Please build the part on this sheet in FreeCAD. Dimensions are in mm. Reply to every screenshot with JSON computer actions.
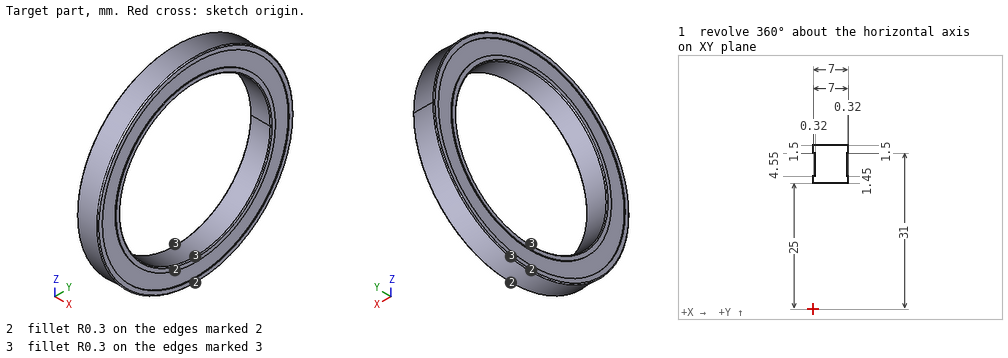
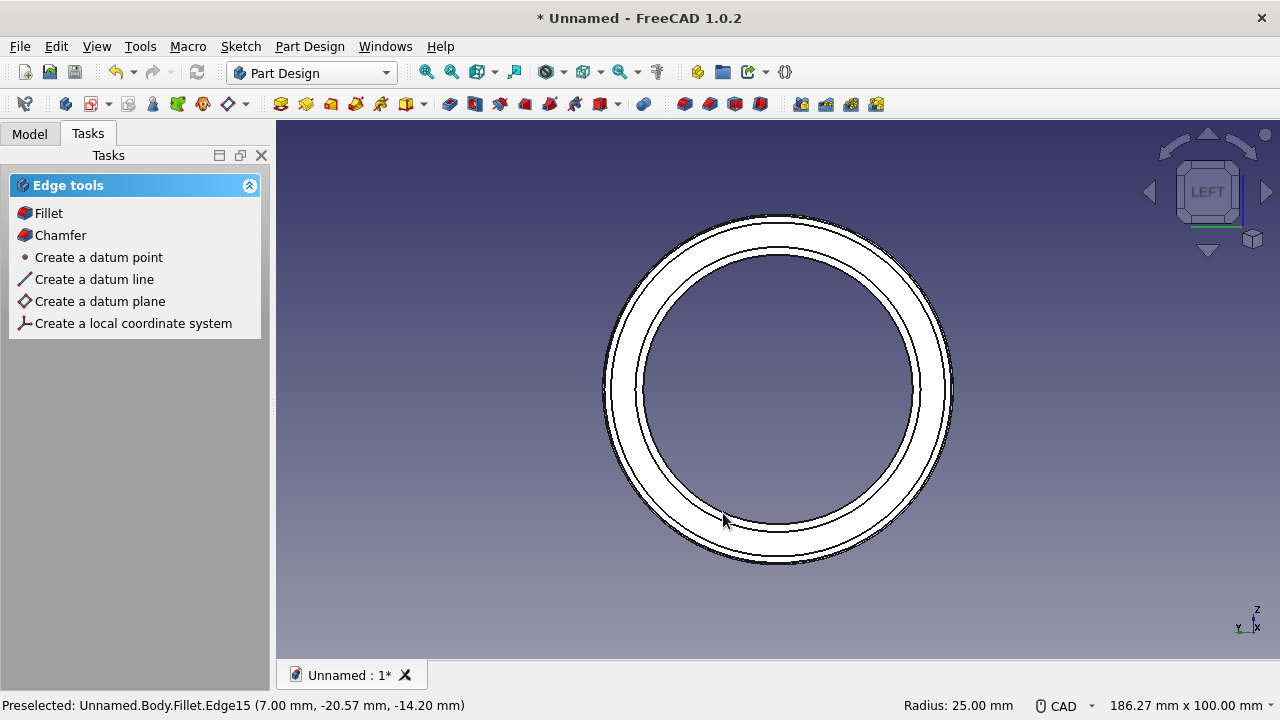
{"action": "left_click", "coordinate": [887, 309], "text": "ctrl"}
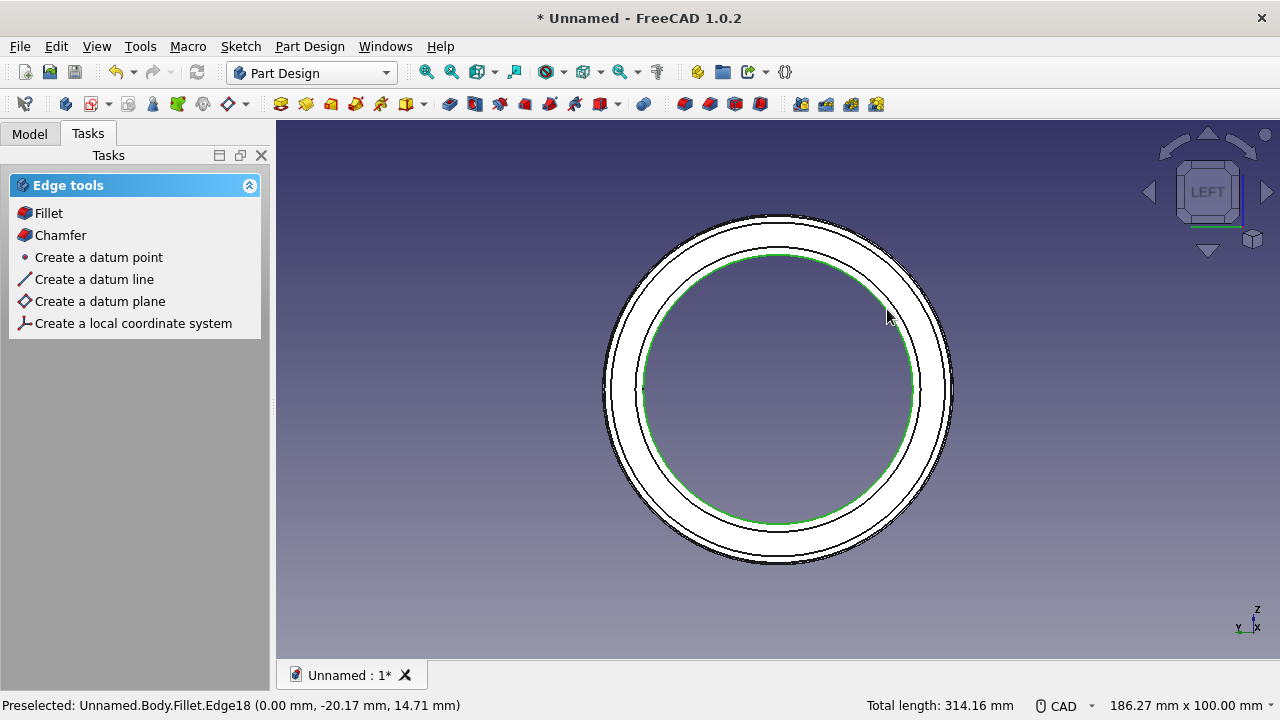
{"action": "left_click", "coordinate": [685, 104]}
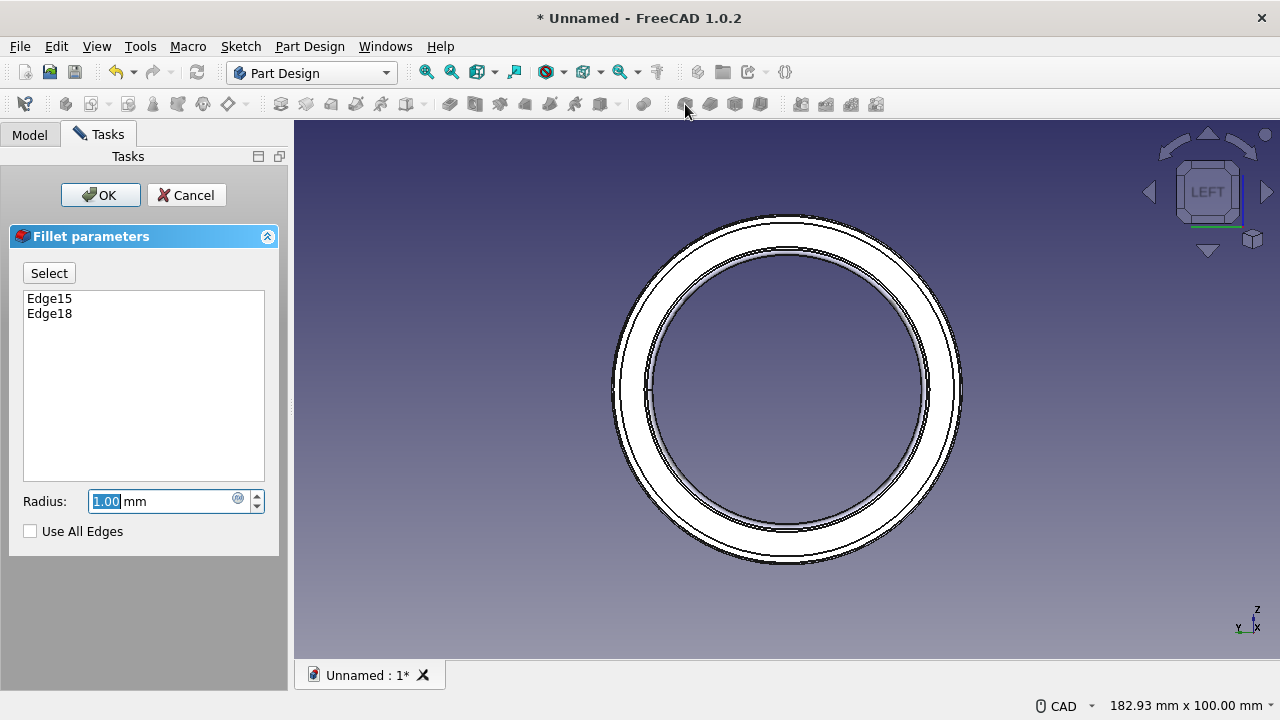
{"action": "type", "text": "0.3"}
{"action": "key", "text": "Tab"}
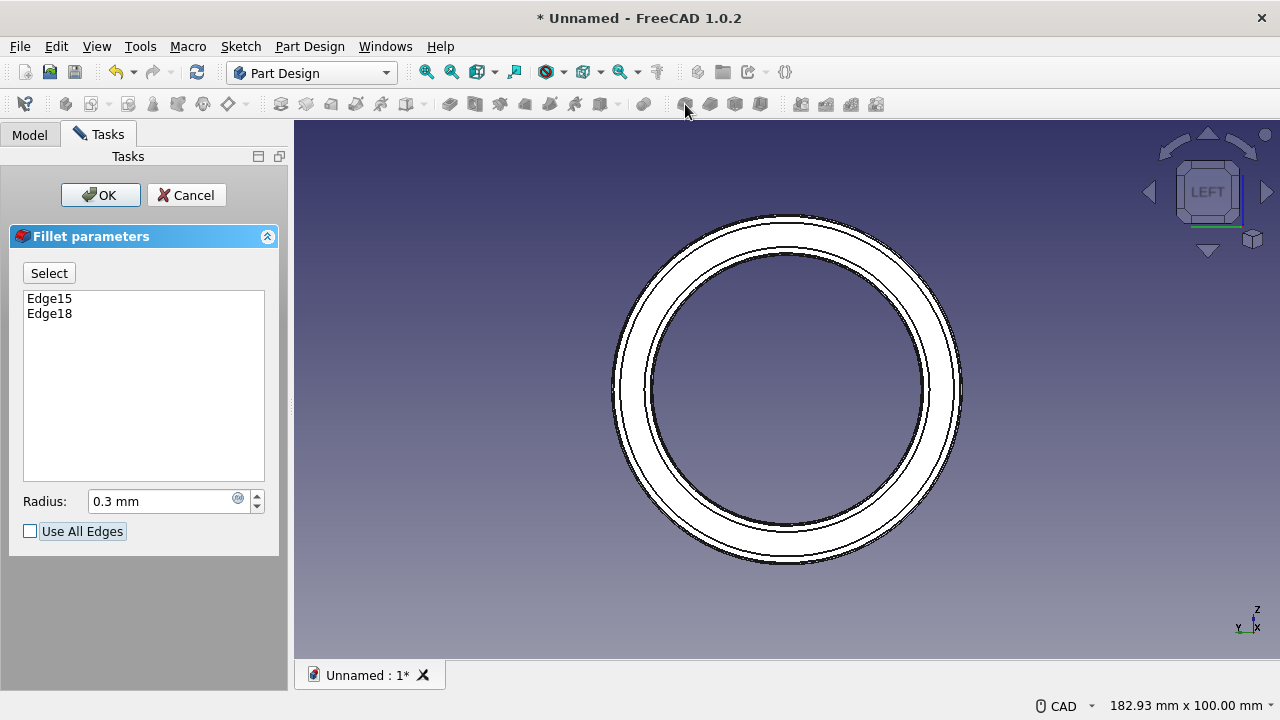
{"action": "left_click", "coordinate": [101, 195]}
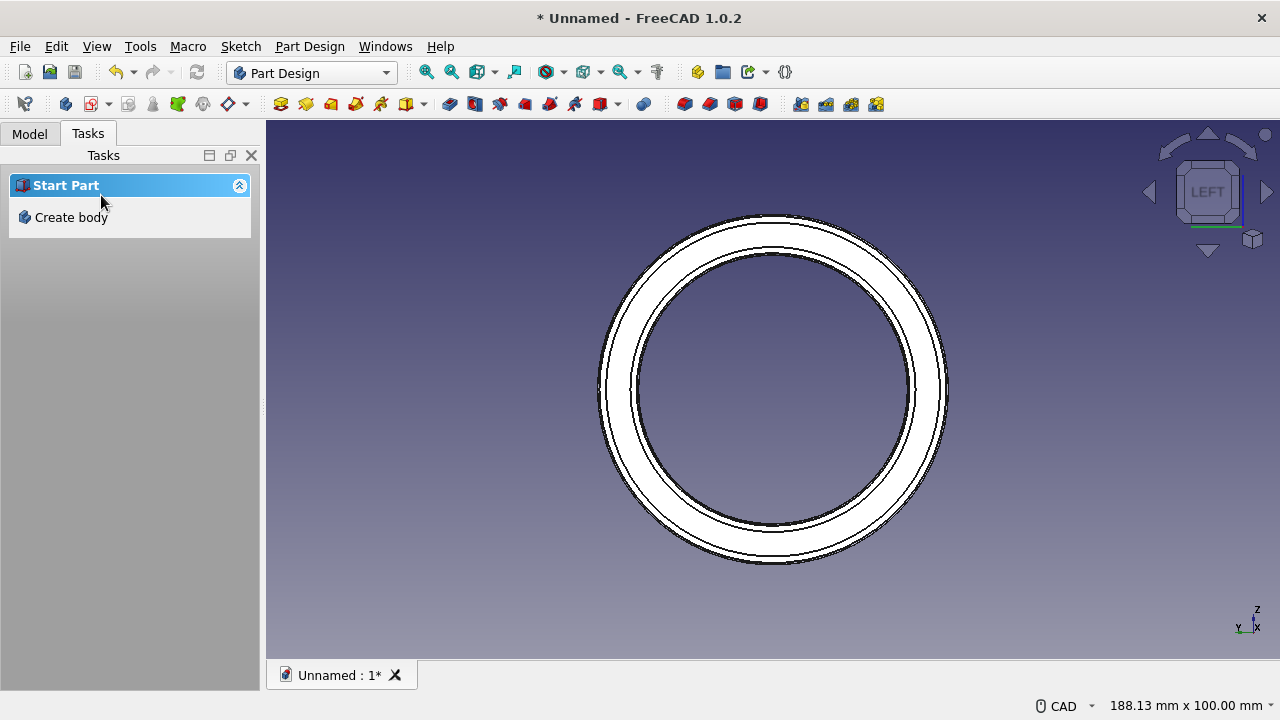
{"action": "key", "text": "0"}